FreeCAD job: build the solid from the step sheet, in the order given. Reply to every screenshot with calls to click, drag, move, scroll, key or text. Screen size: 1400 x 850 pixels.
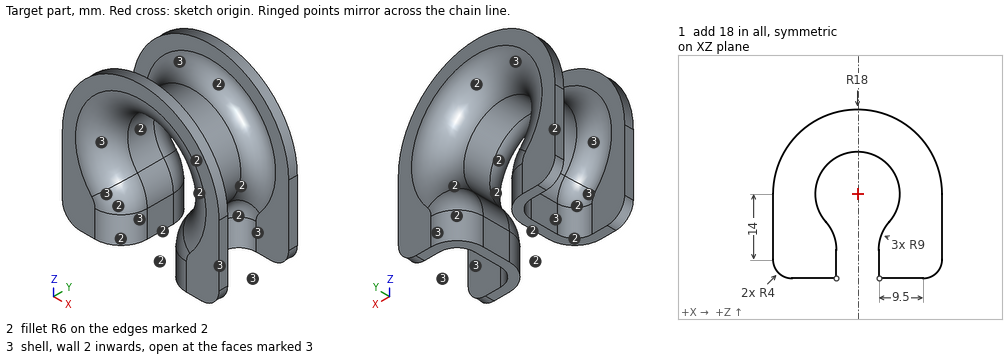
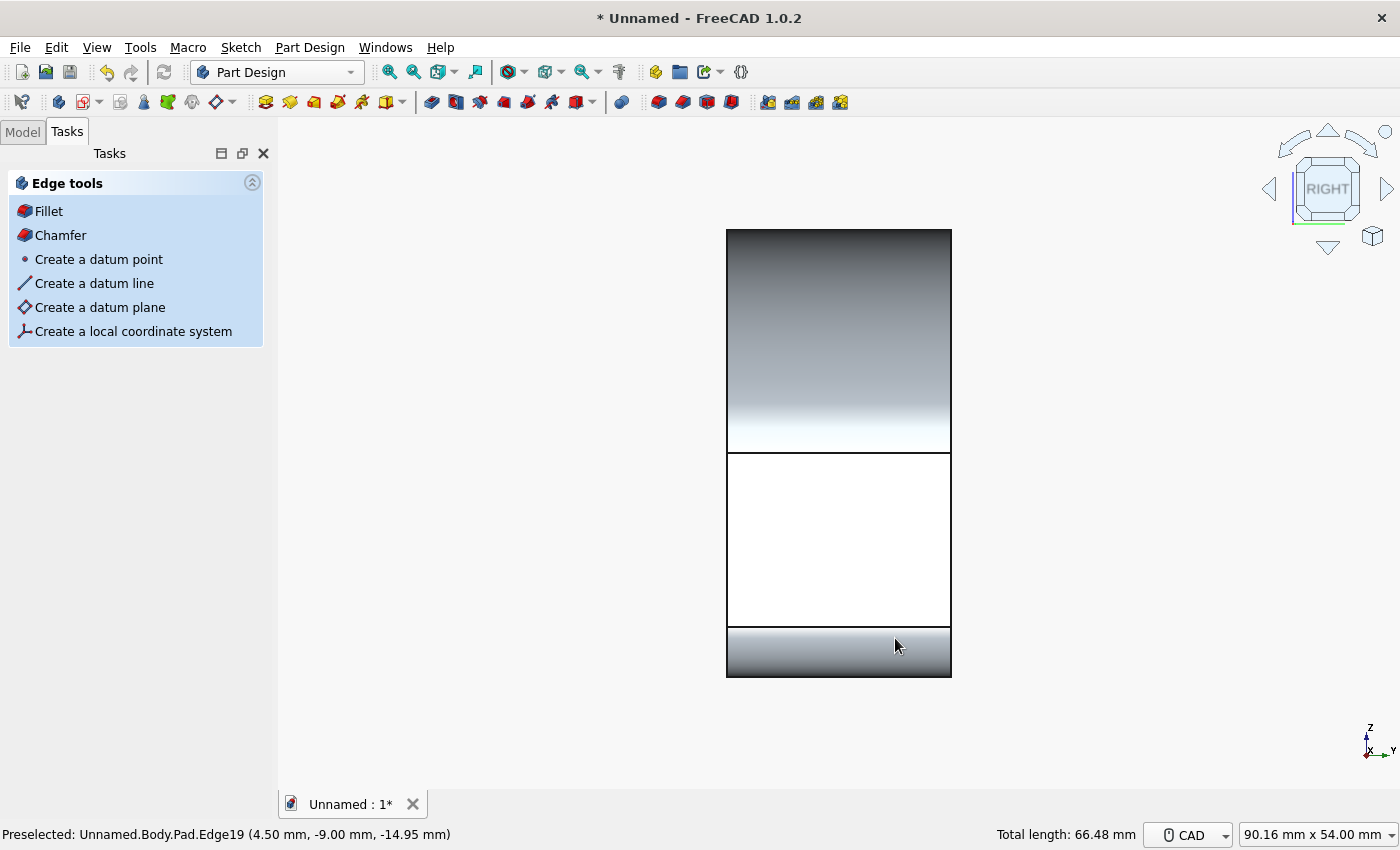
key(5)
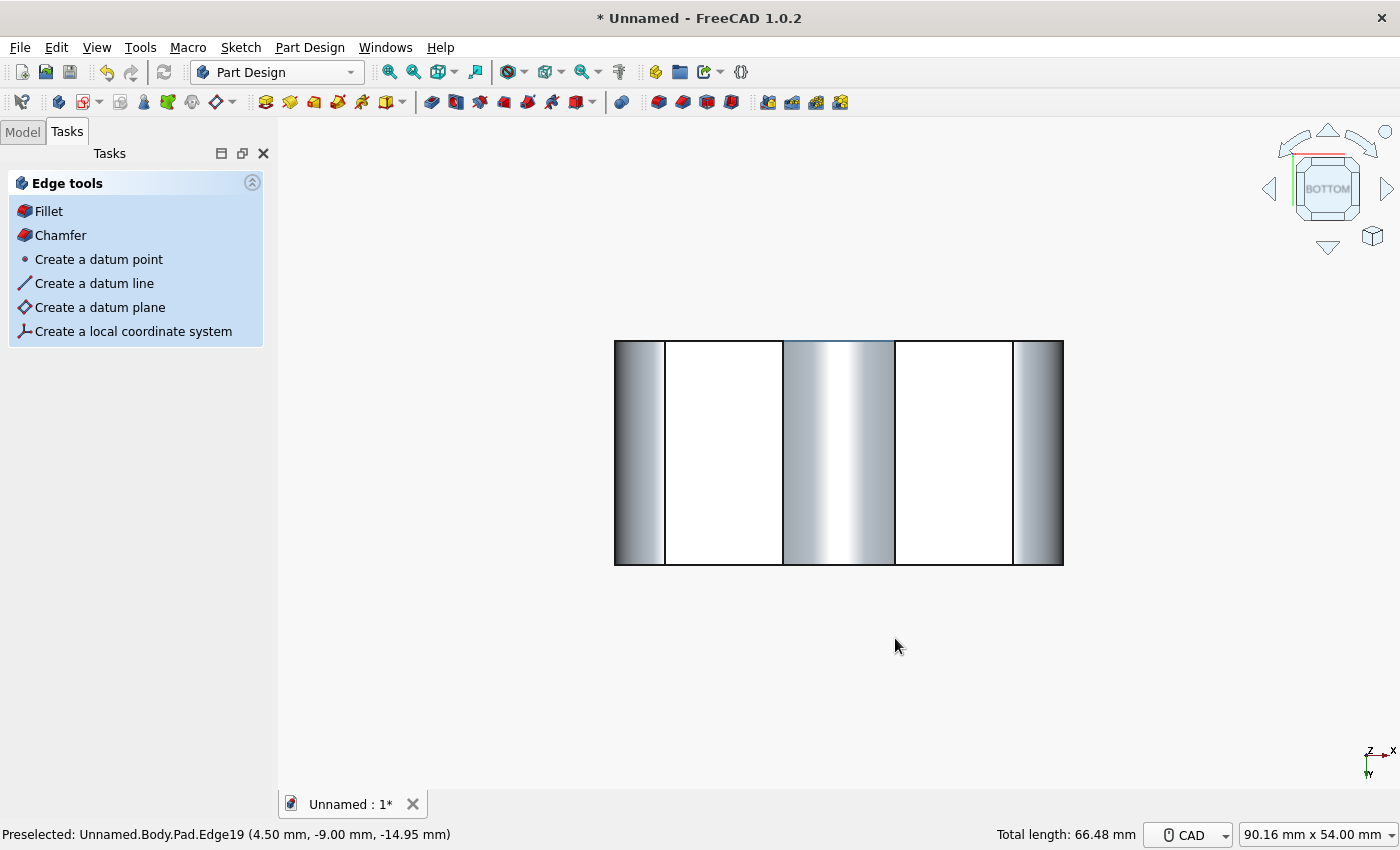
click(390, 72)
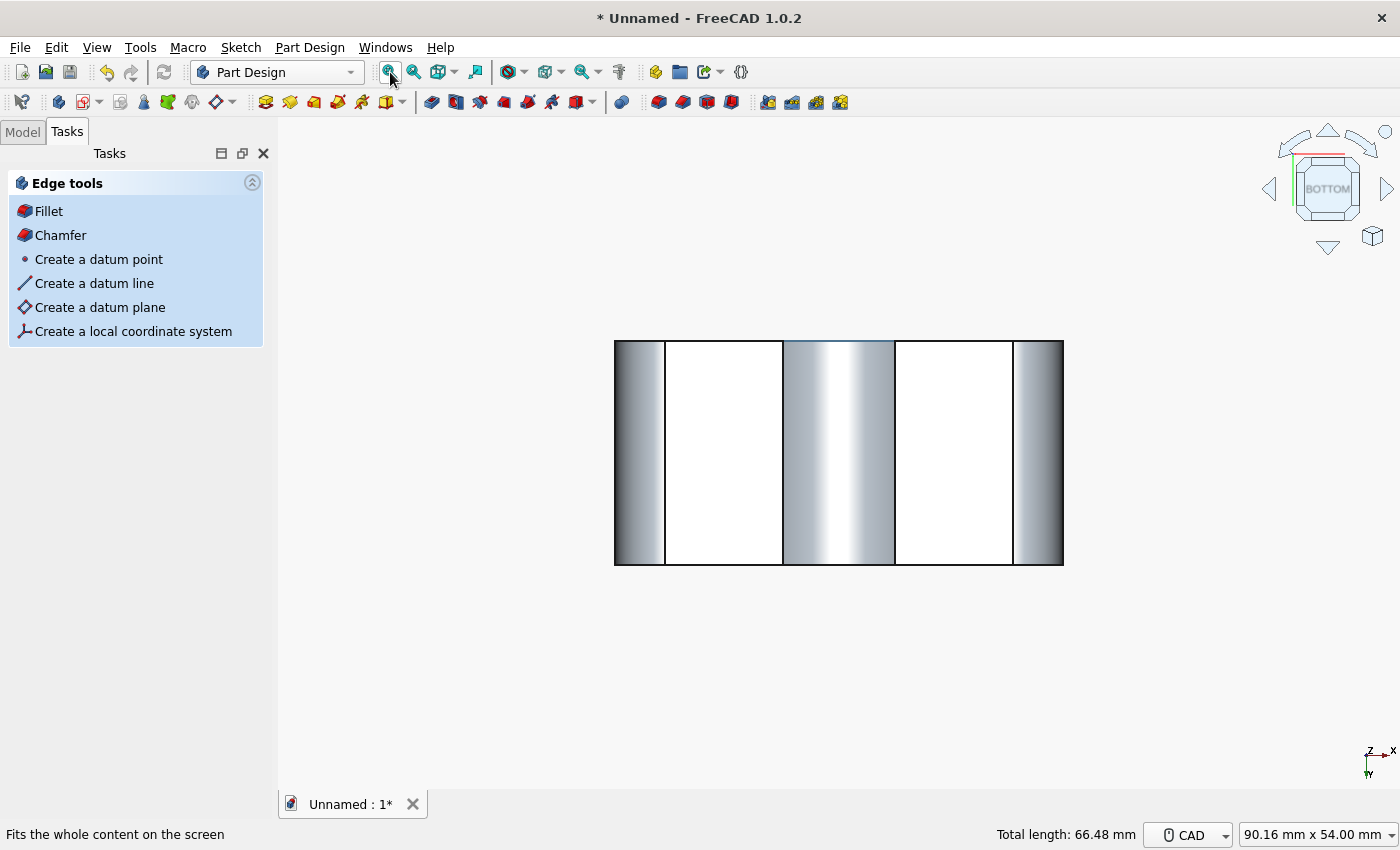
key(4)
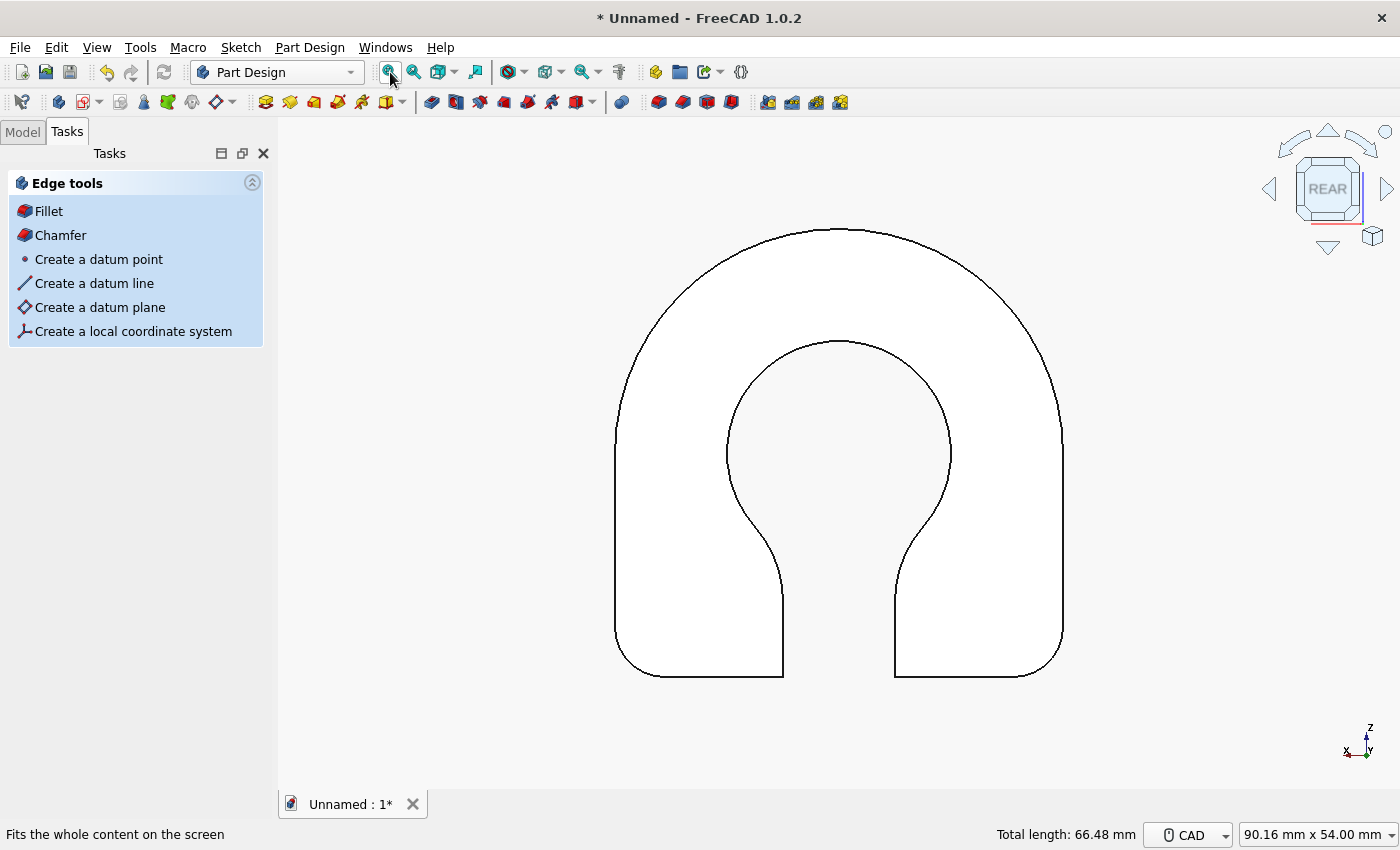
click(783, 638, ctrl)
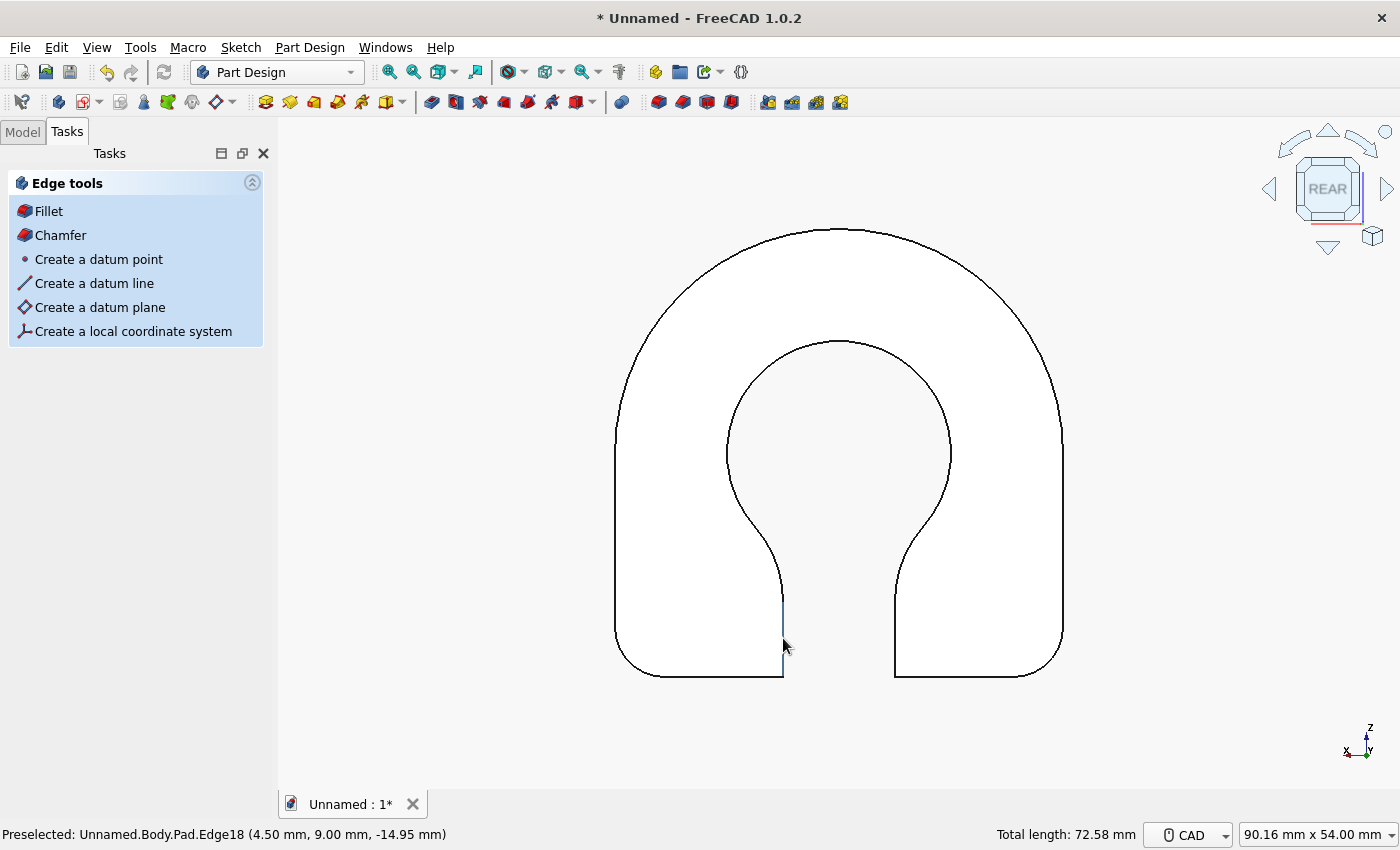
click(839, 340, ctrl)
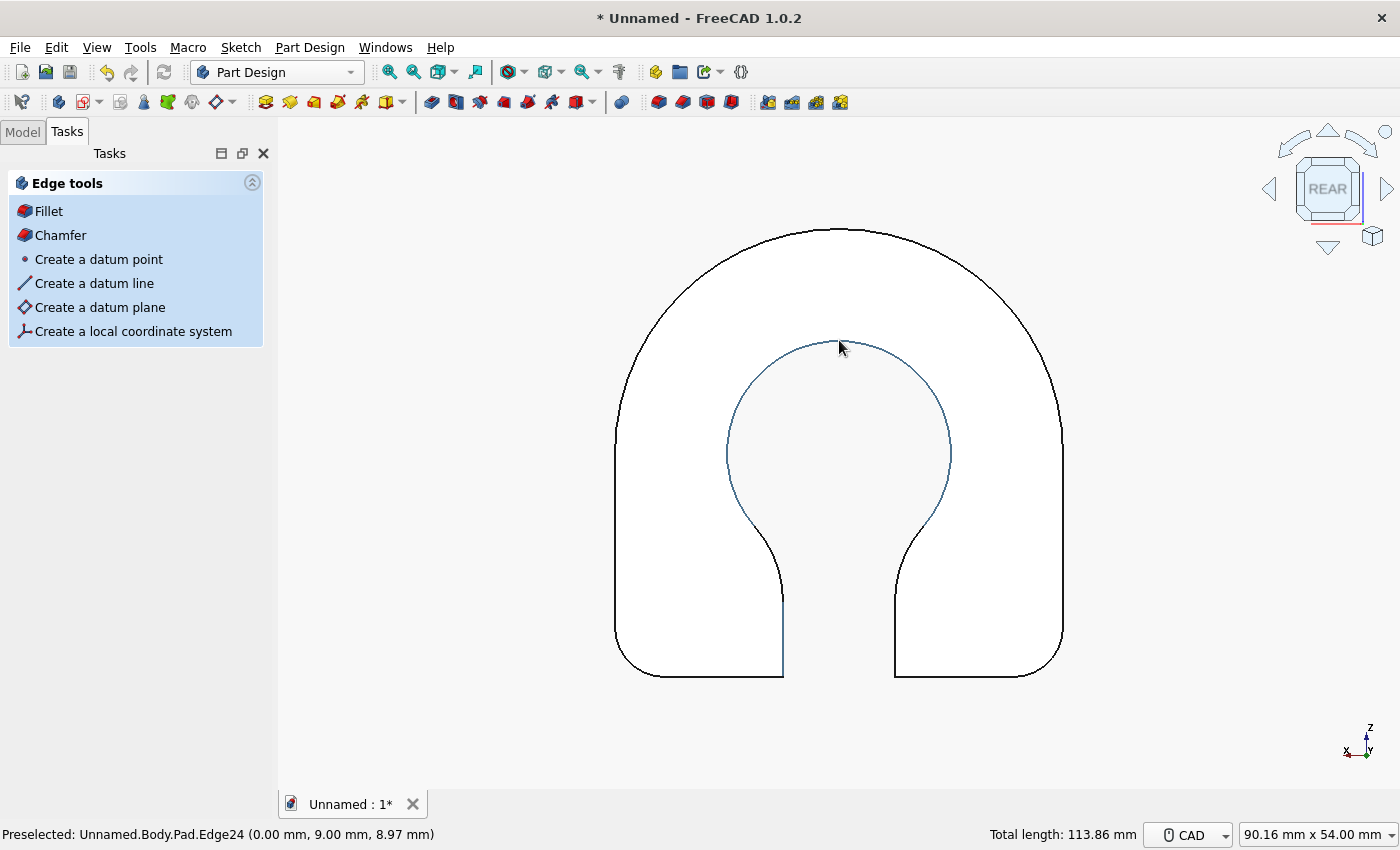
click(895, 638, ctrl)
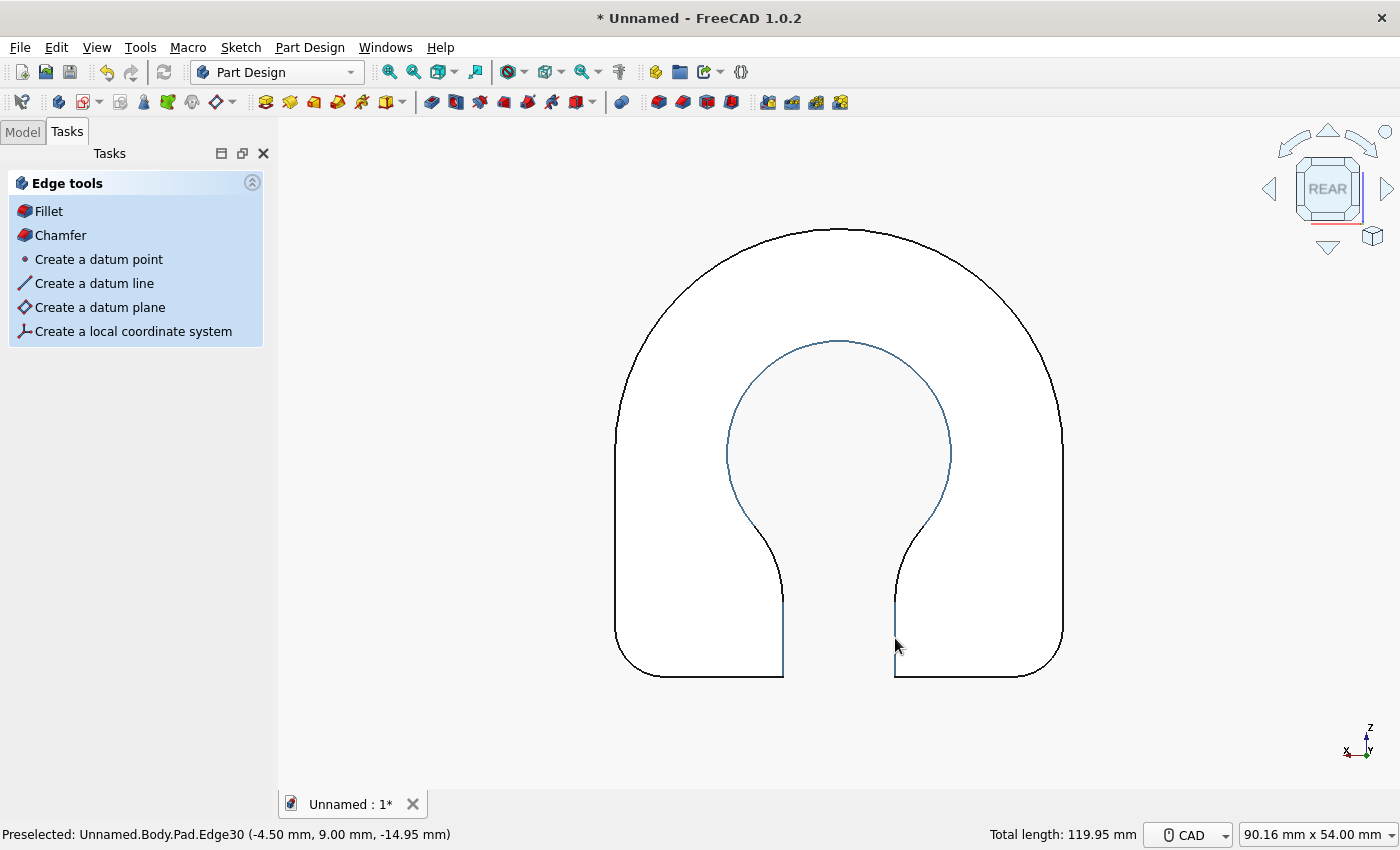
key(6)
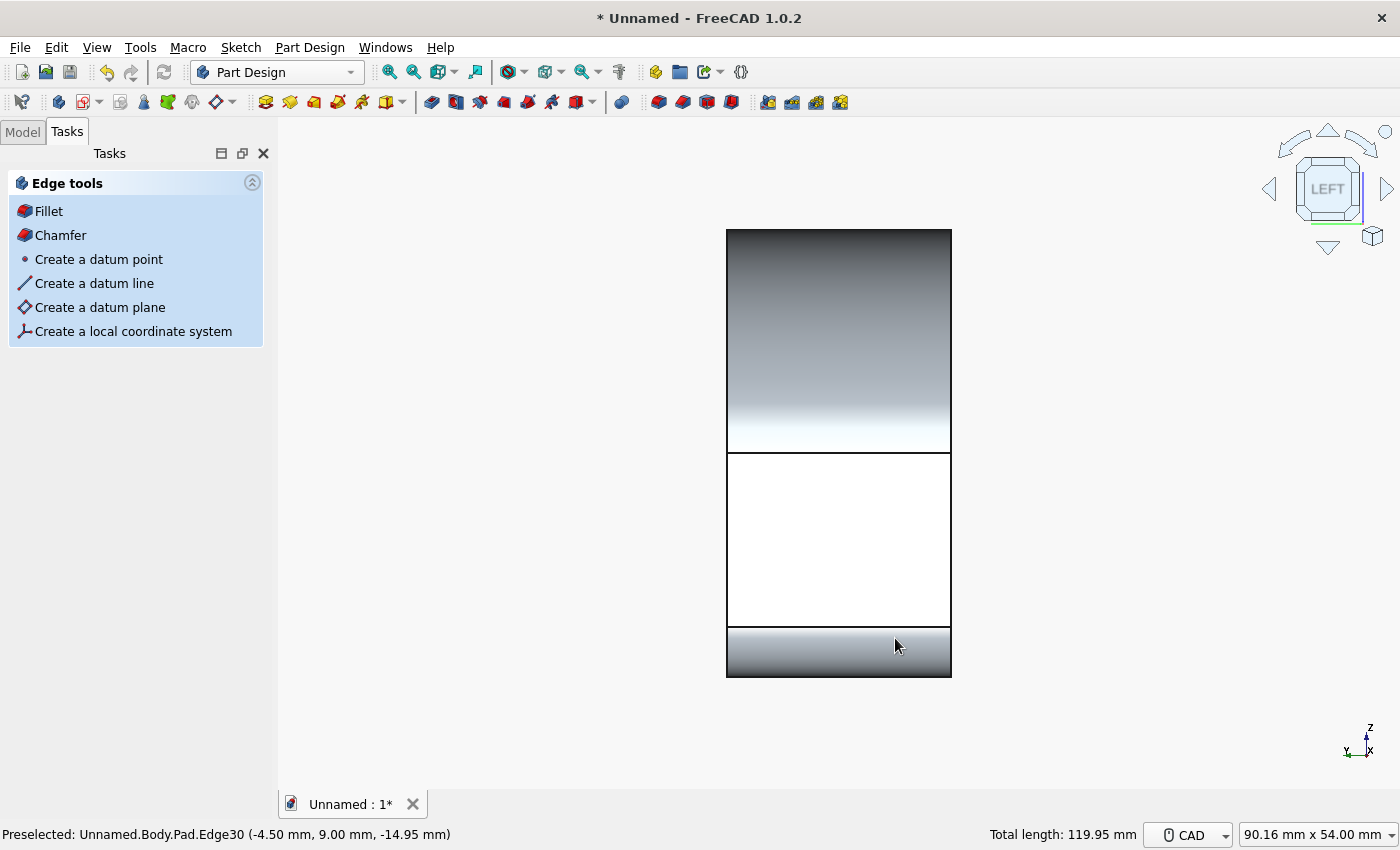
key(v)
key(3)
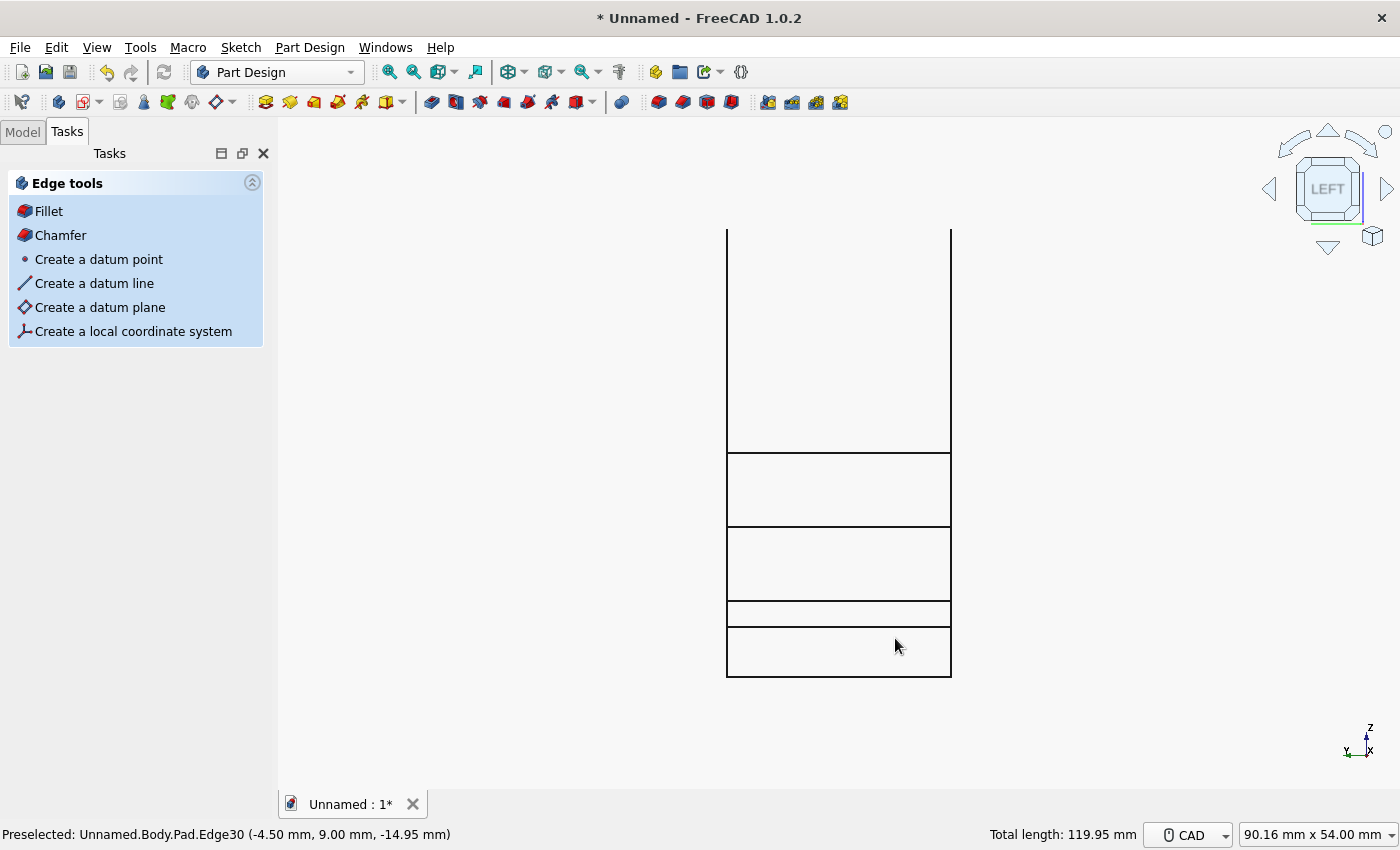
key(0)